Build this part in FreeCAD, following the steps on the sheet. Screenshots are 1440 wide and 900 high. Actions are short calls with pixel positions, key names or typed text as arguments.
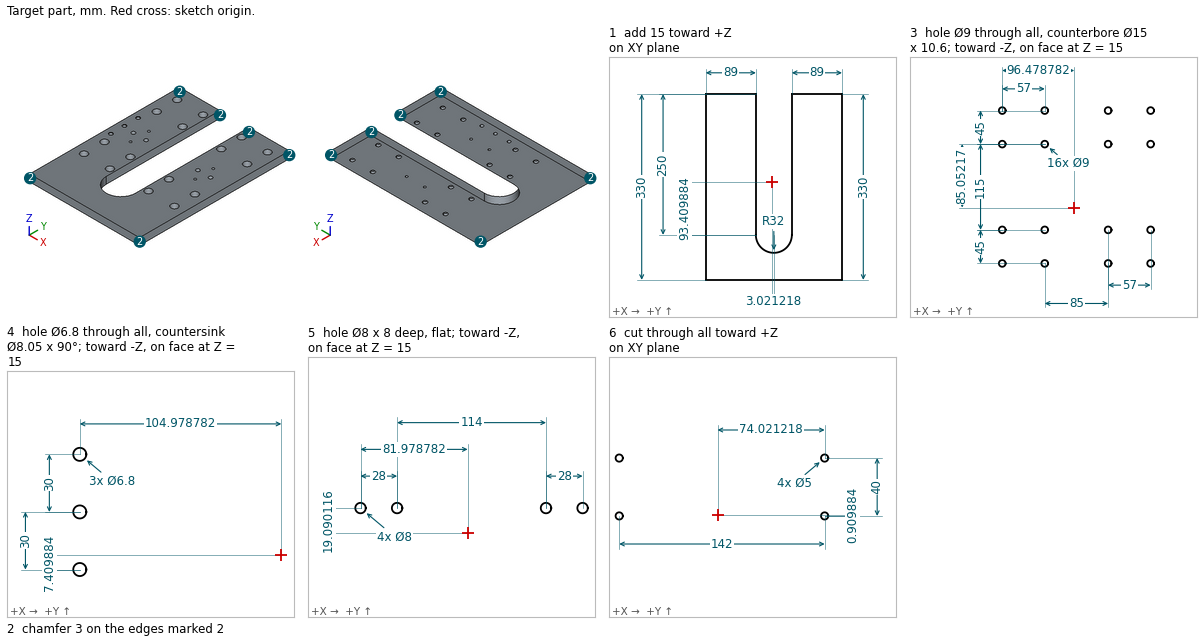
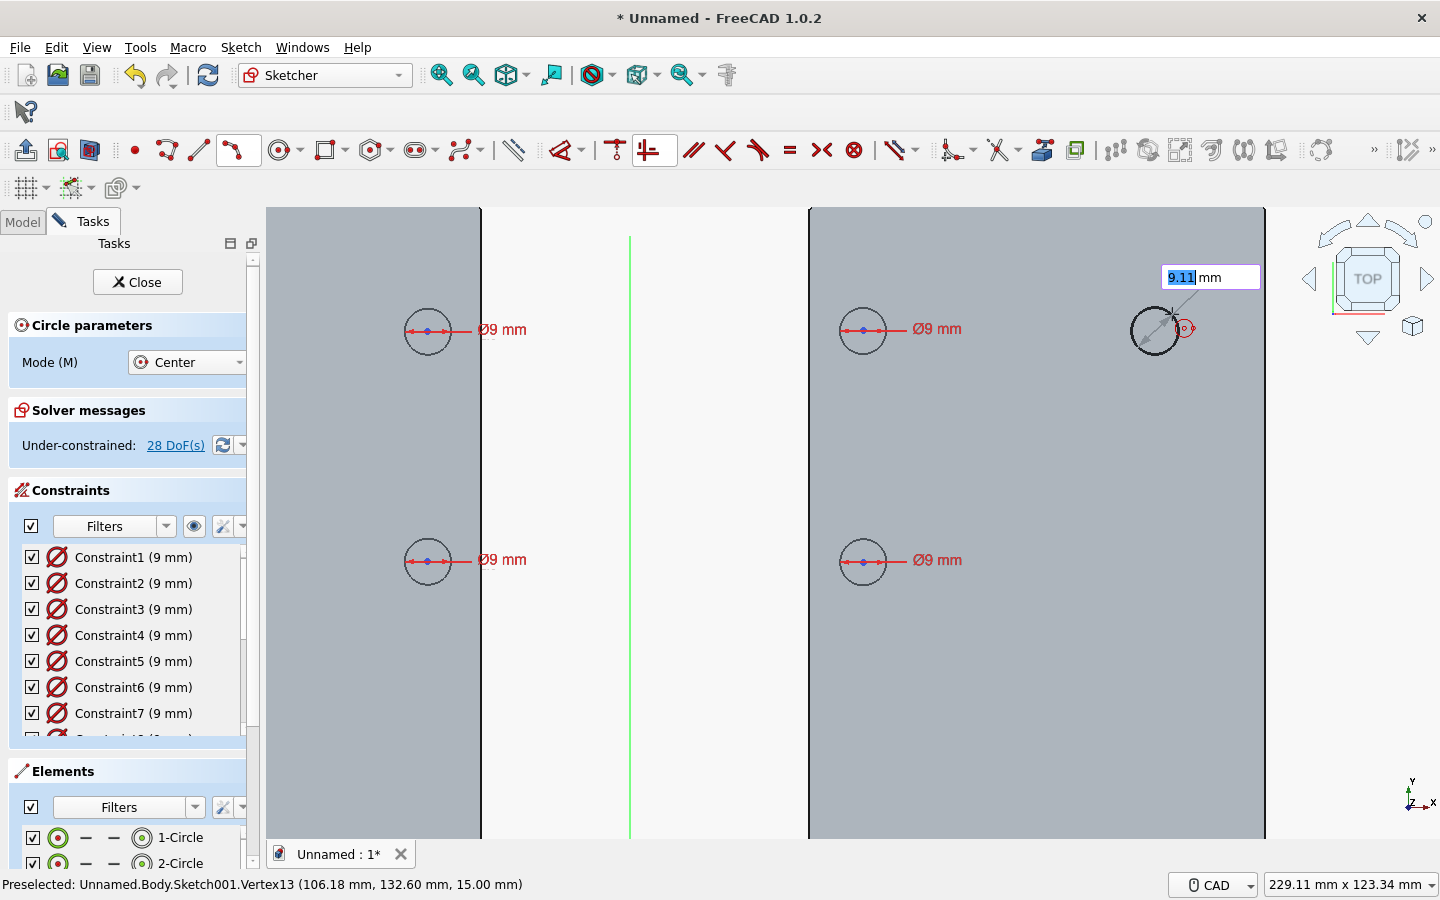
text(9)
key(Return)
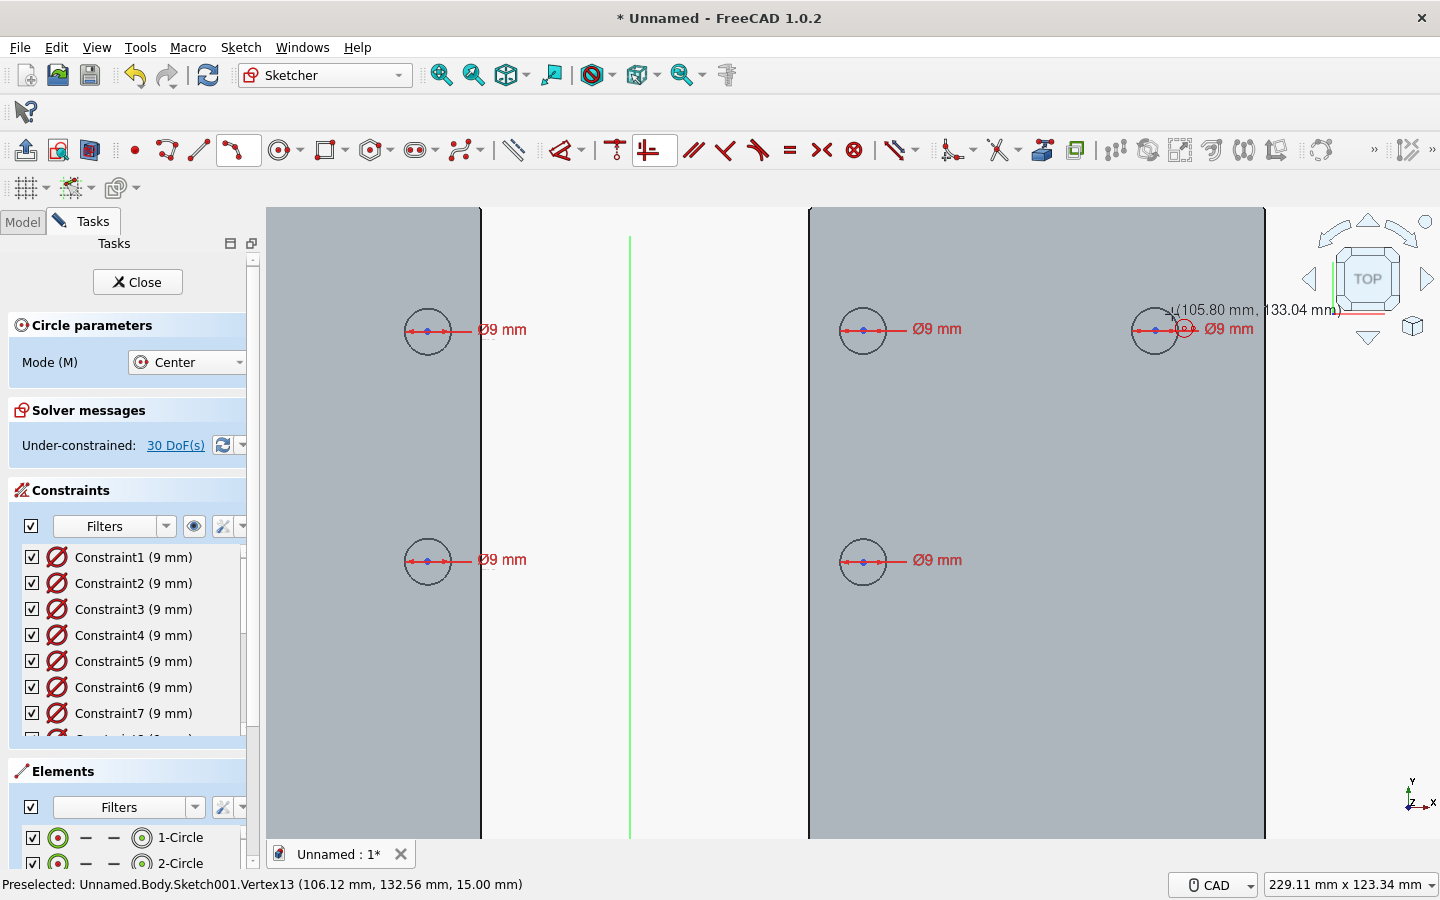
click(1155, 561)
move(1172, 545)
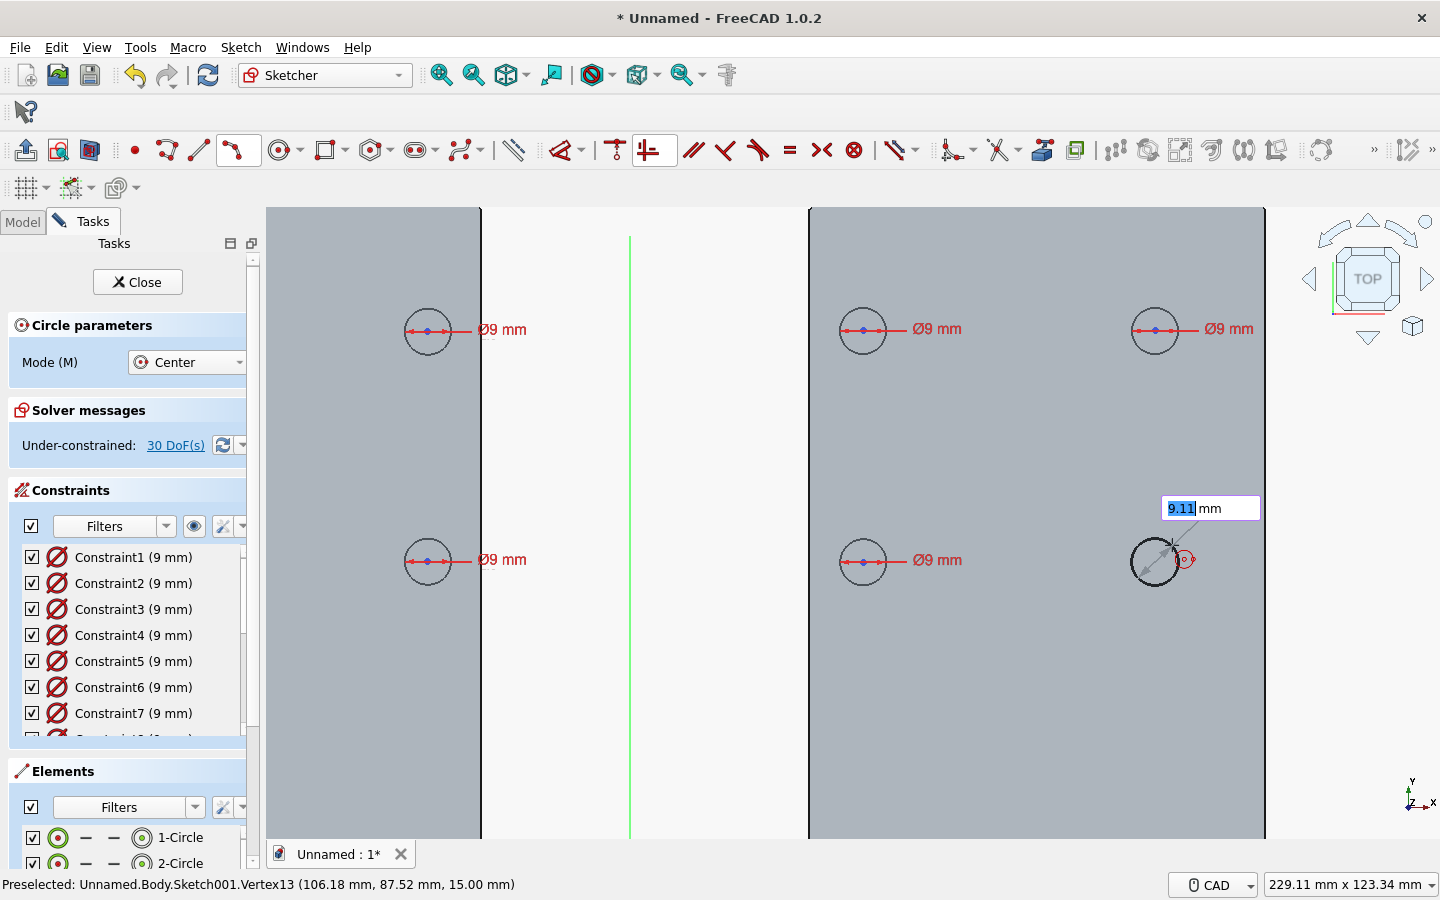
text(9)
key(Return)
key(Escape)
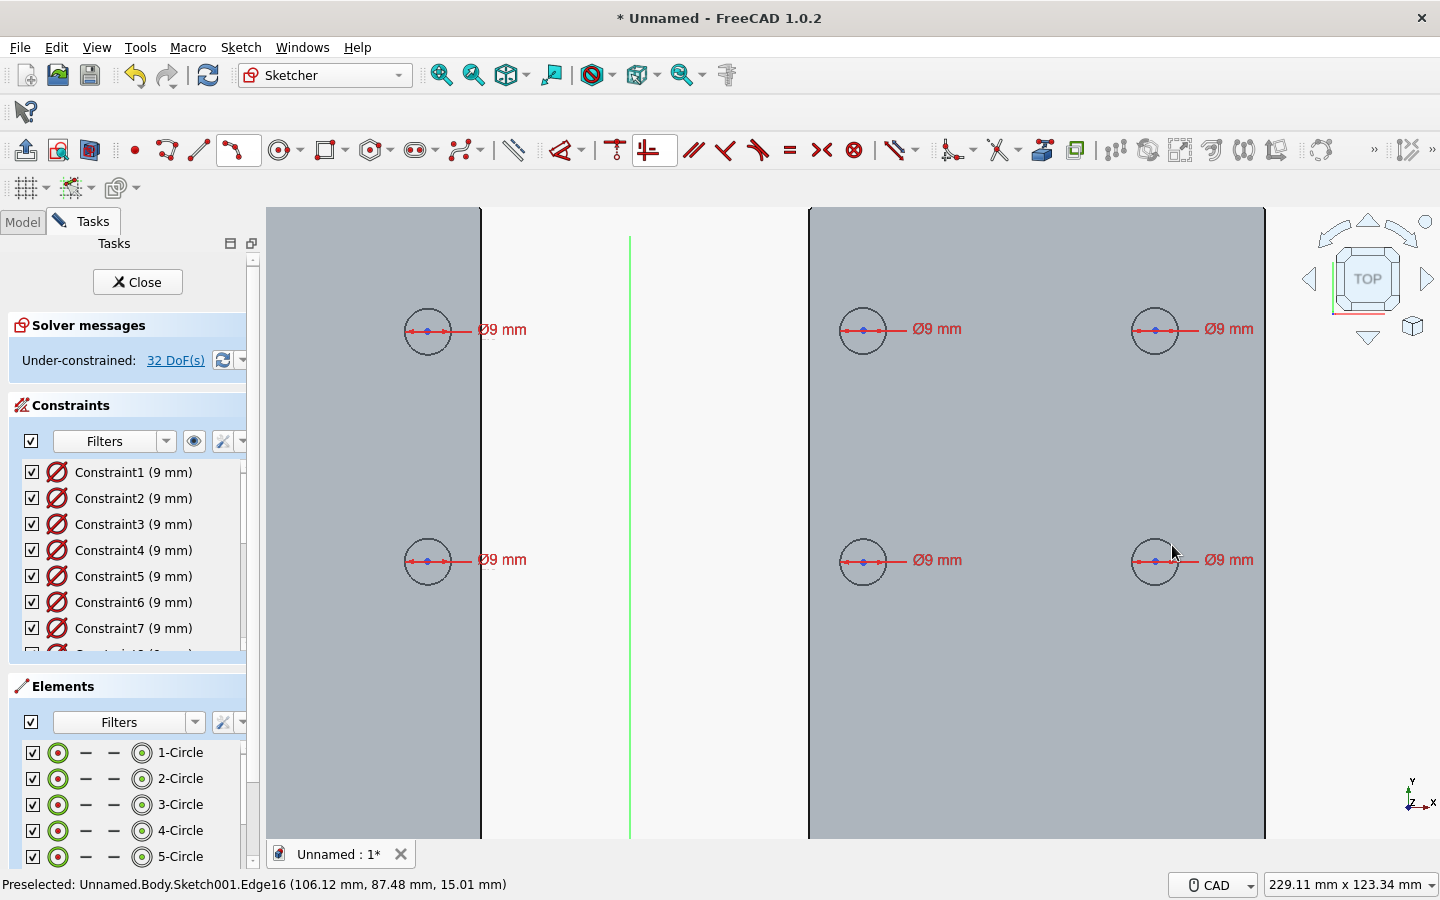
scroll(865, 329, down, 5)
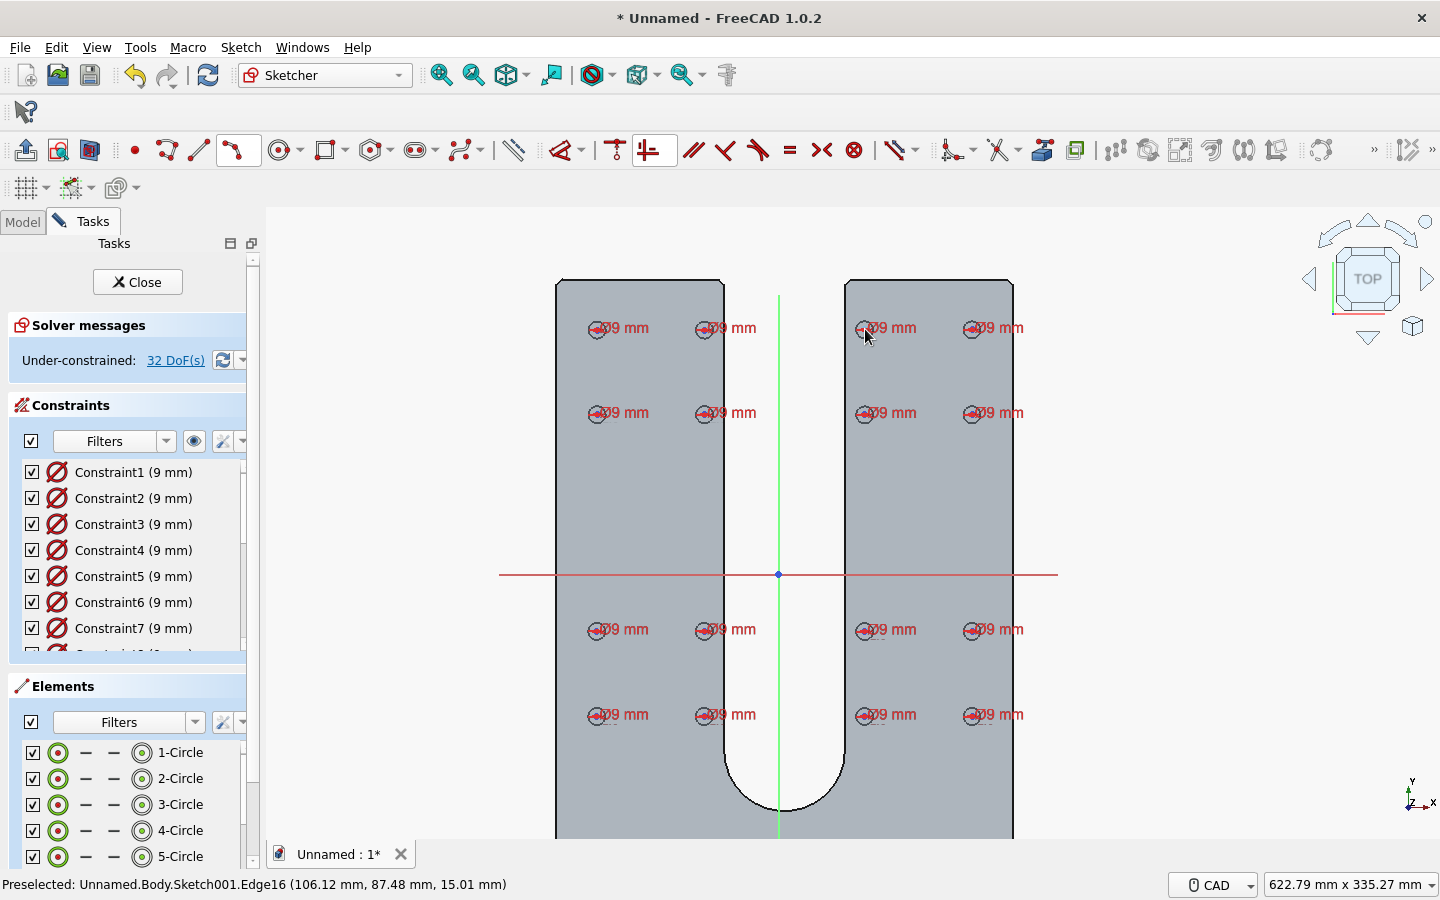
click(597, 330)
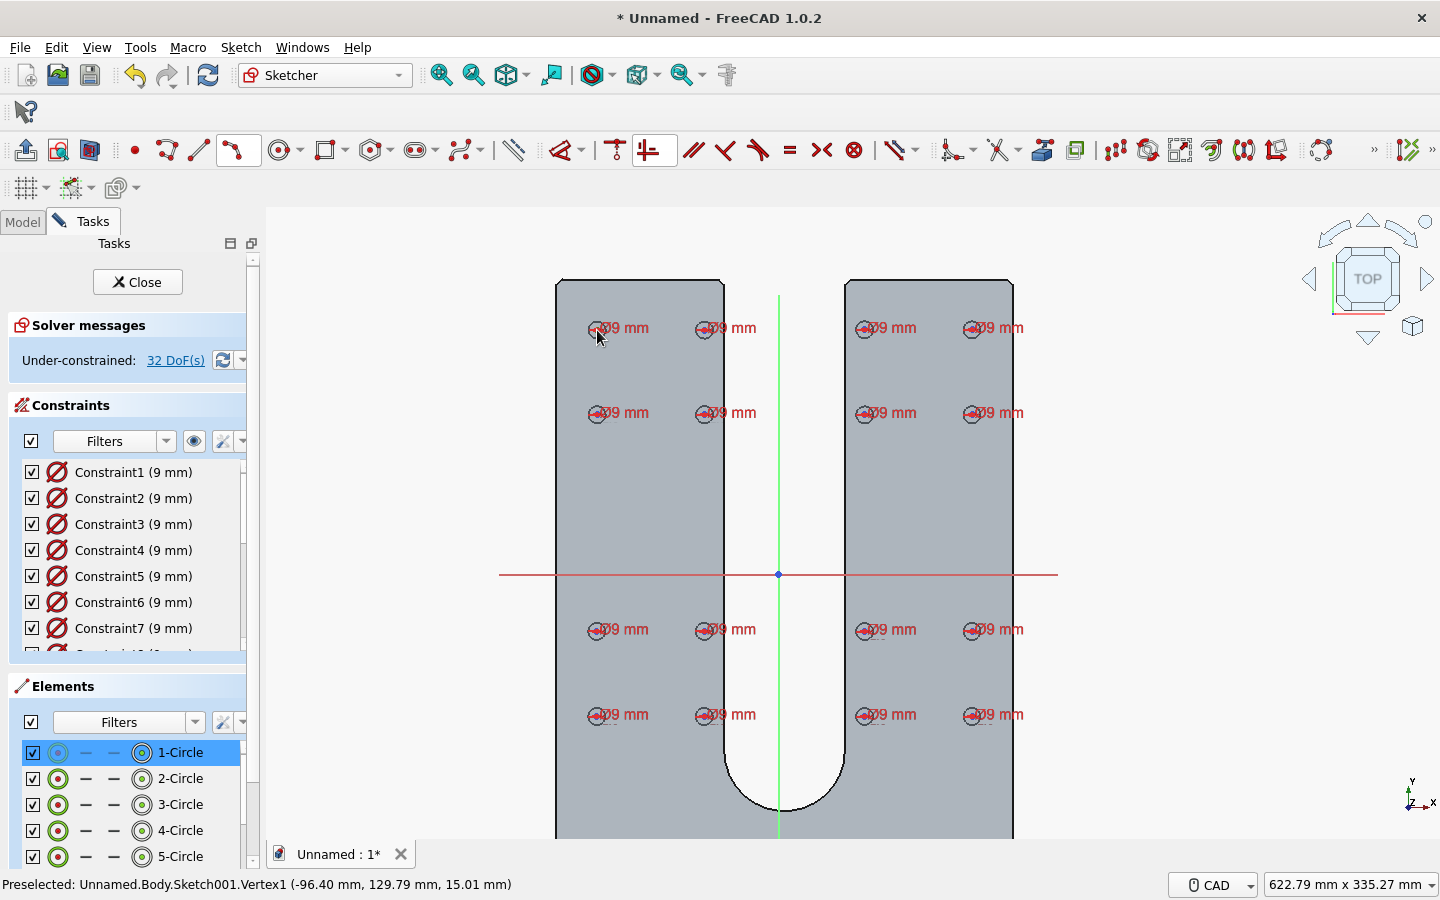
click(705, 330)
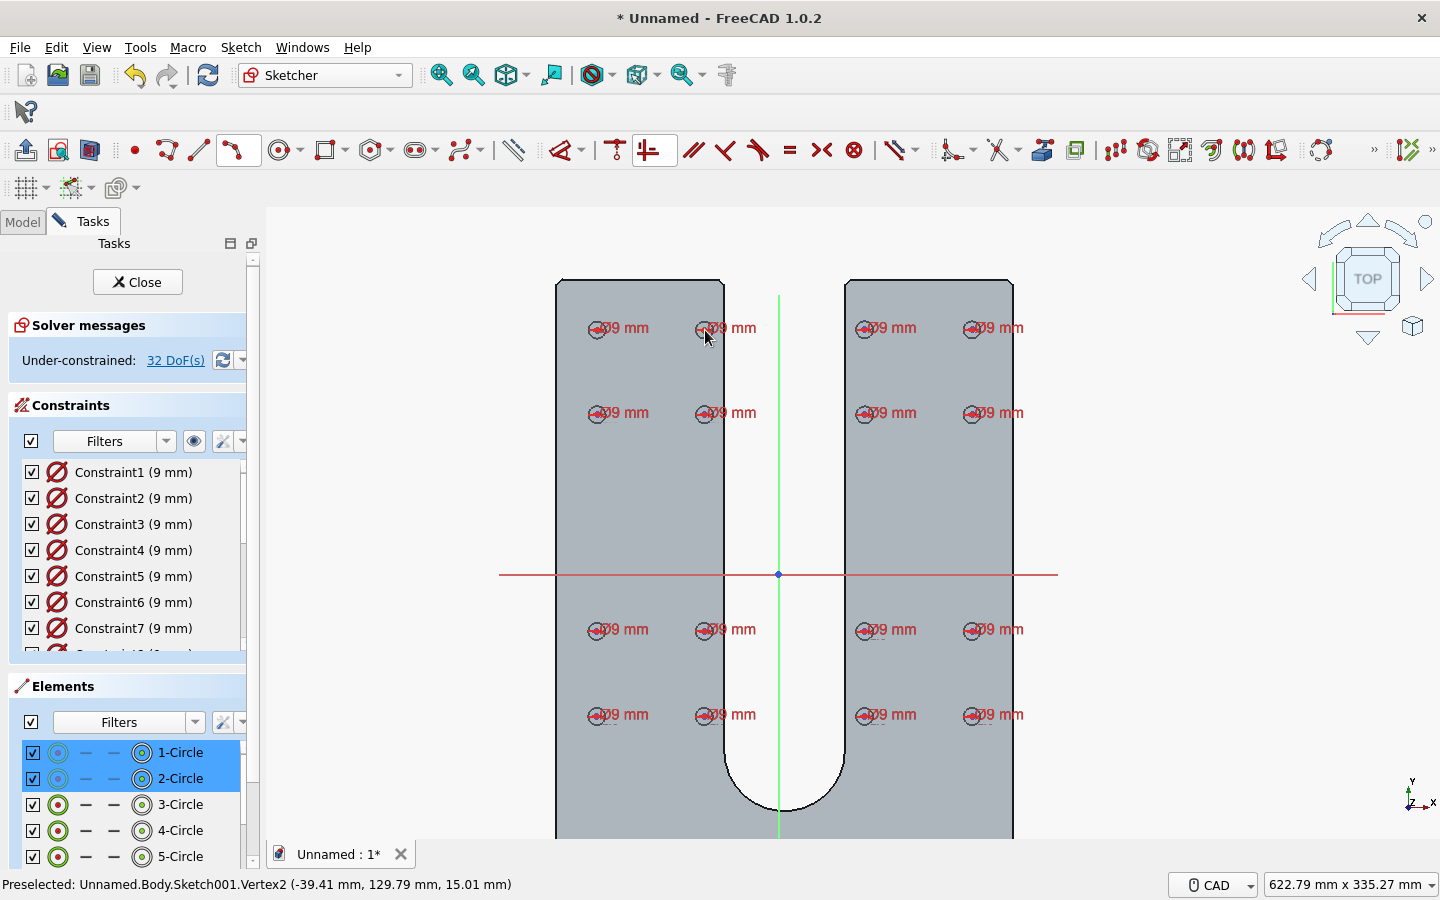
click(672, 150)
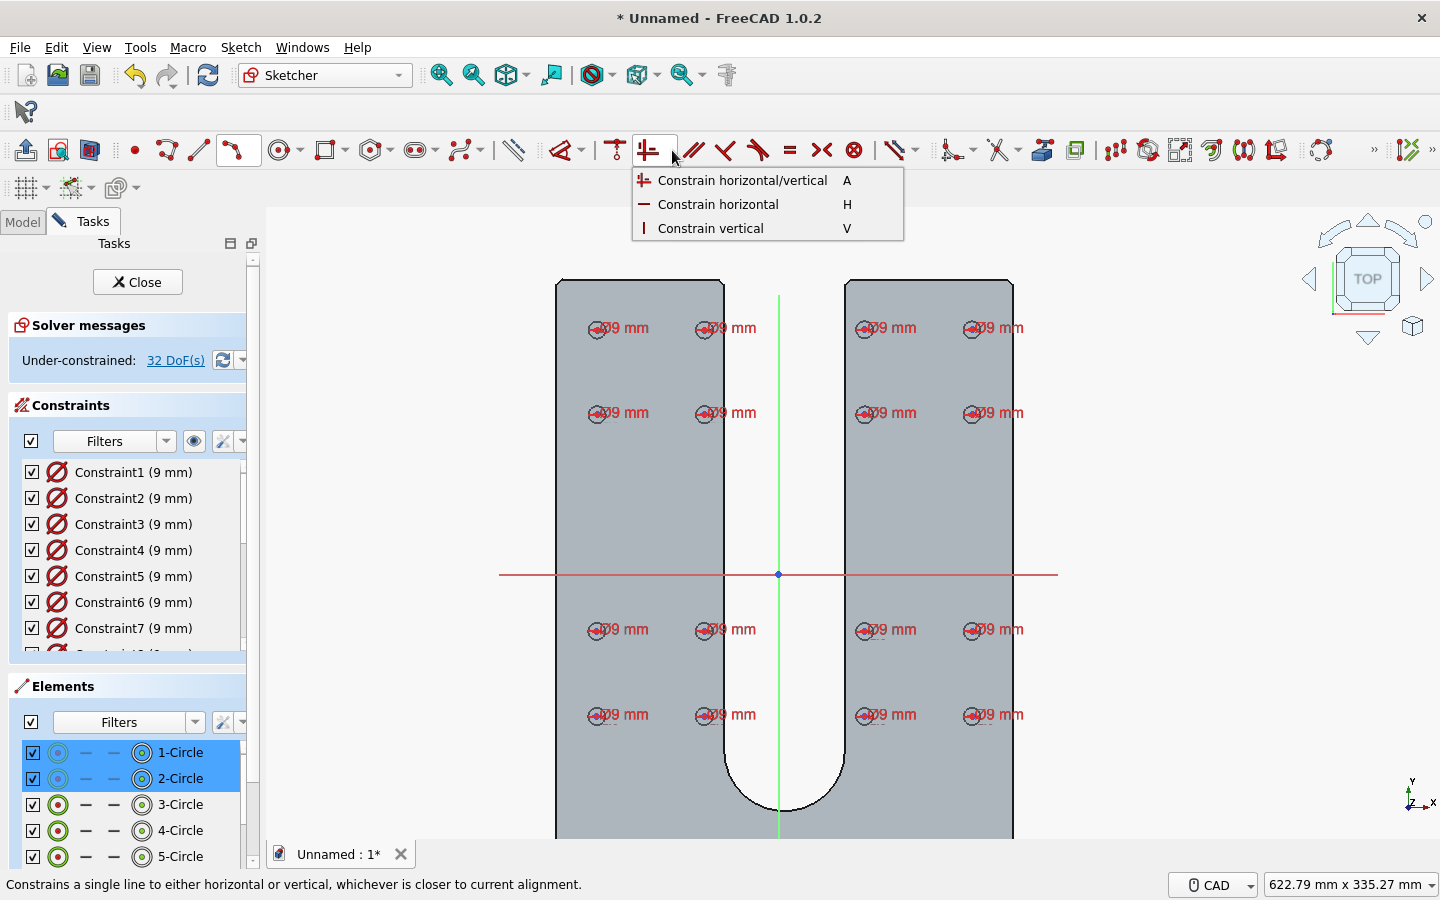
click(768, 204)